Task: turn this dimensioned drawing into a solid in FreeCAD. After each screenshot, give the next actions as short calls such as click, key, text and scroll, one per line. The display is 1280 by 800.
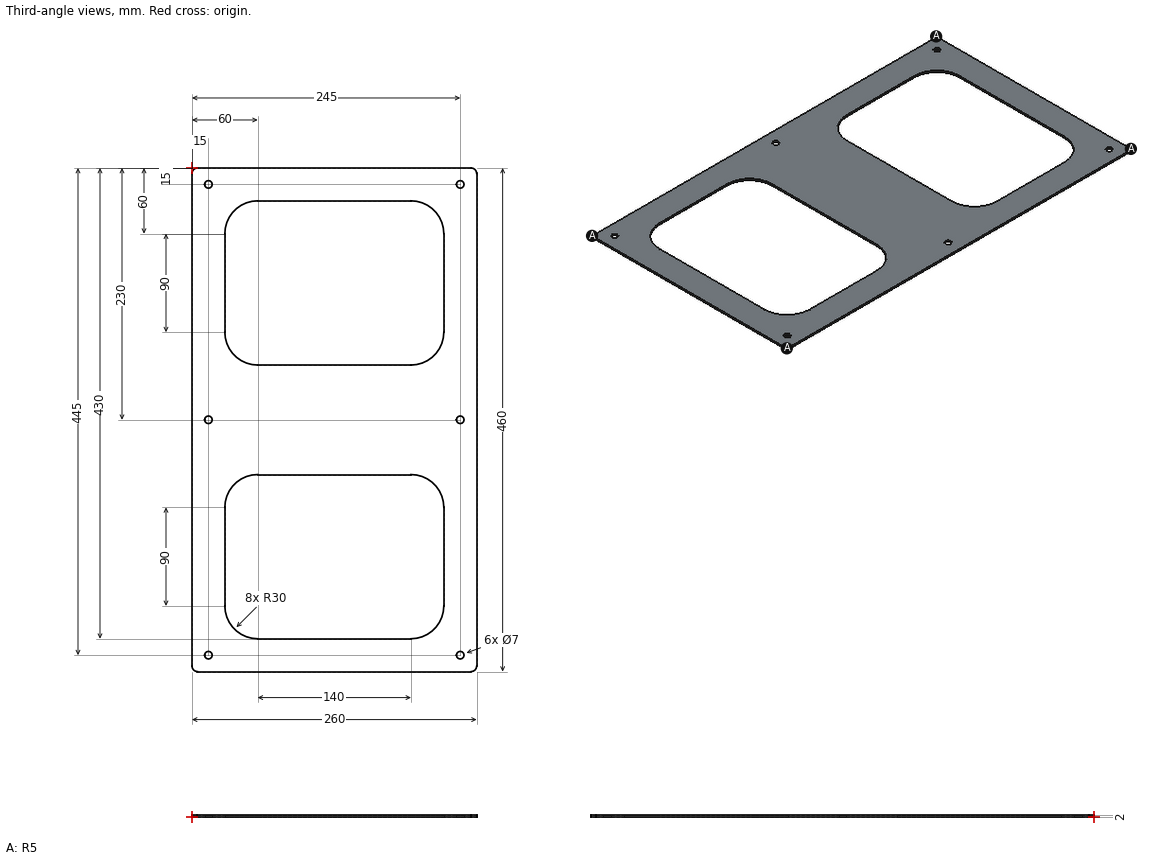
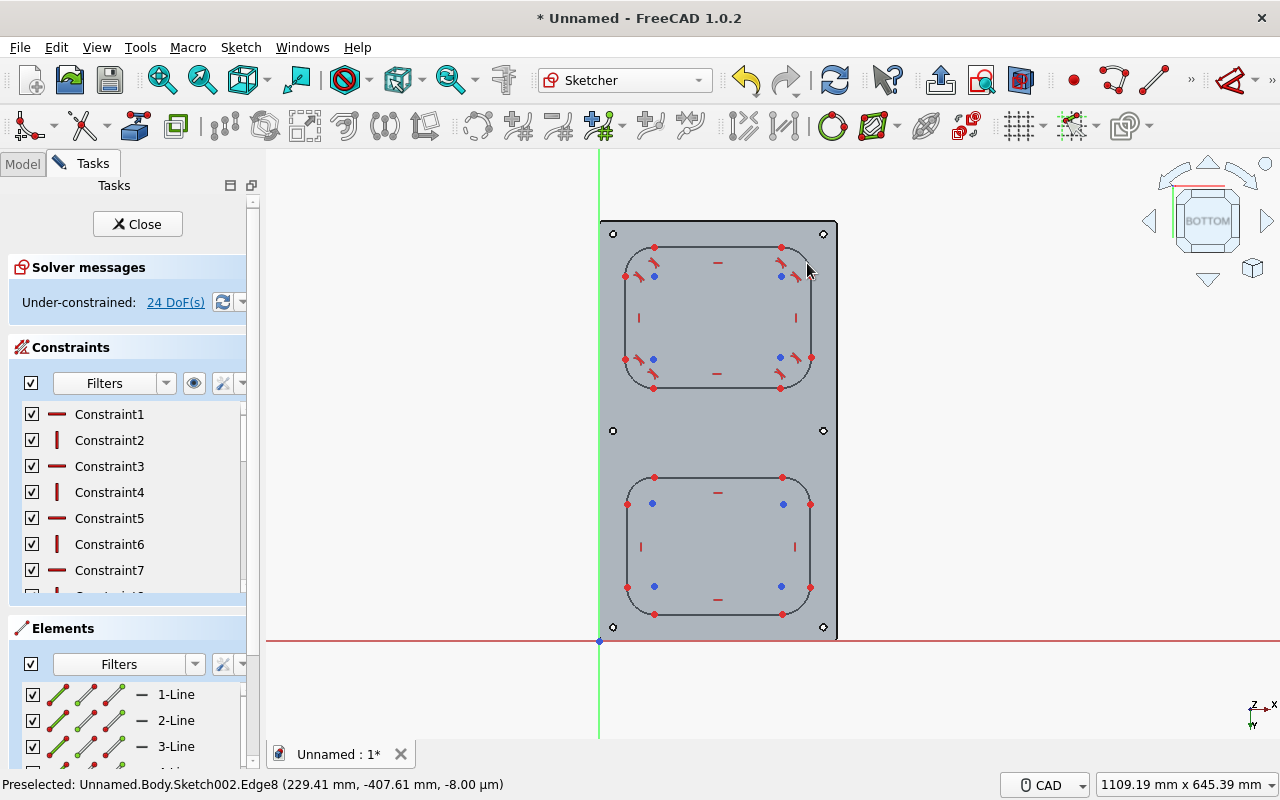
click(744, 478)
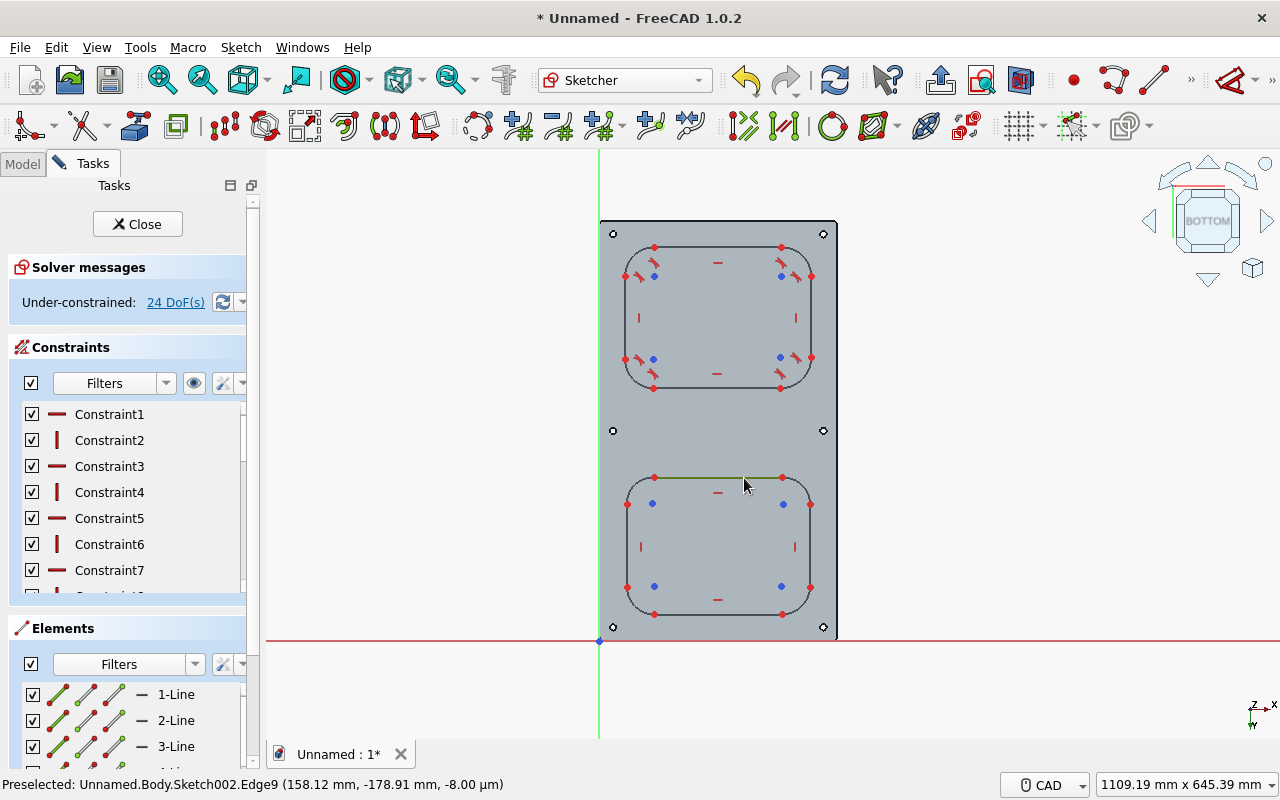
click(642, 480)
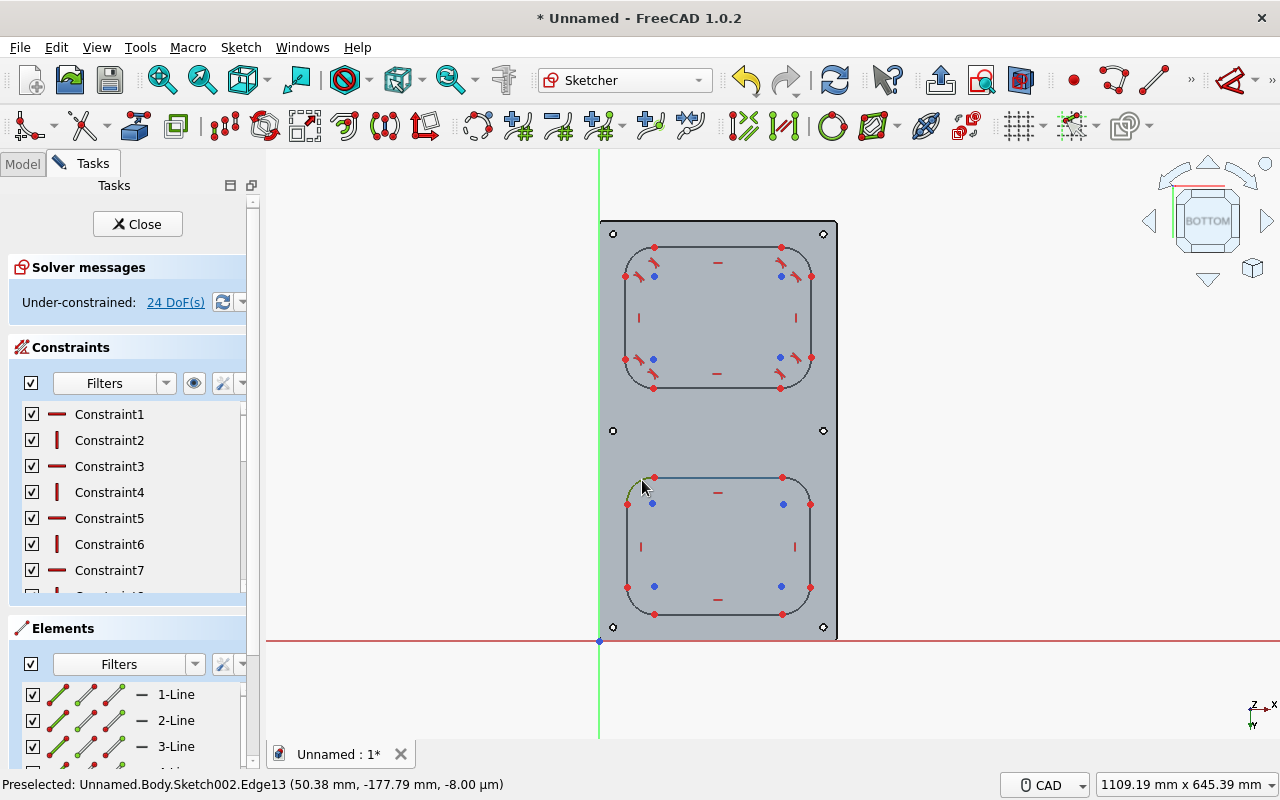
key(t)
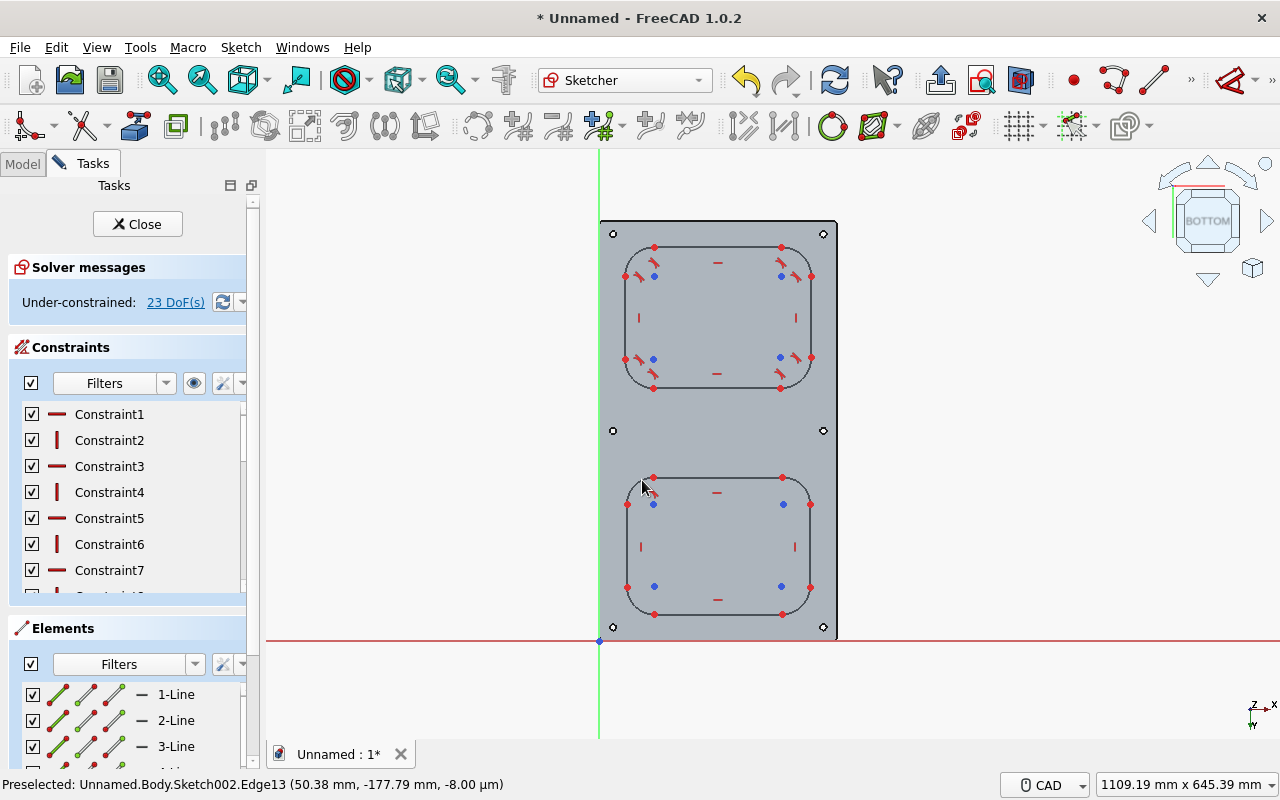
click(744, 478)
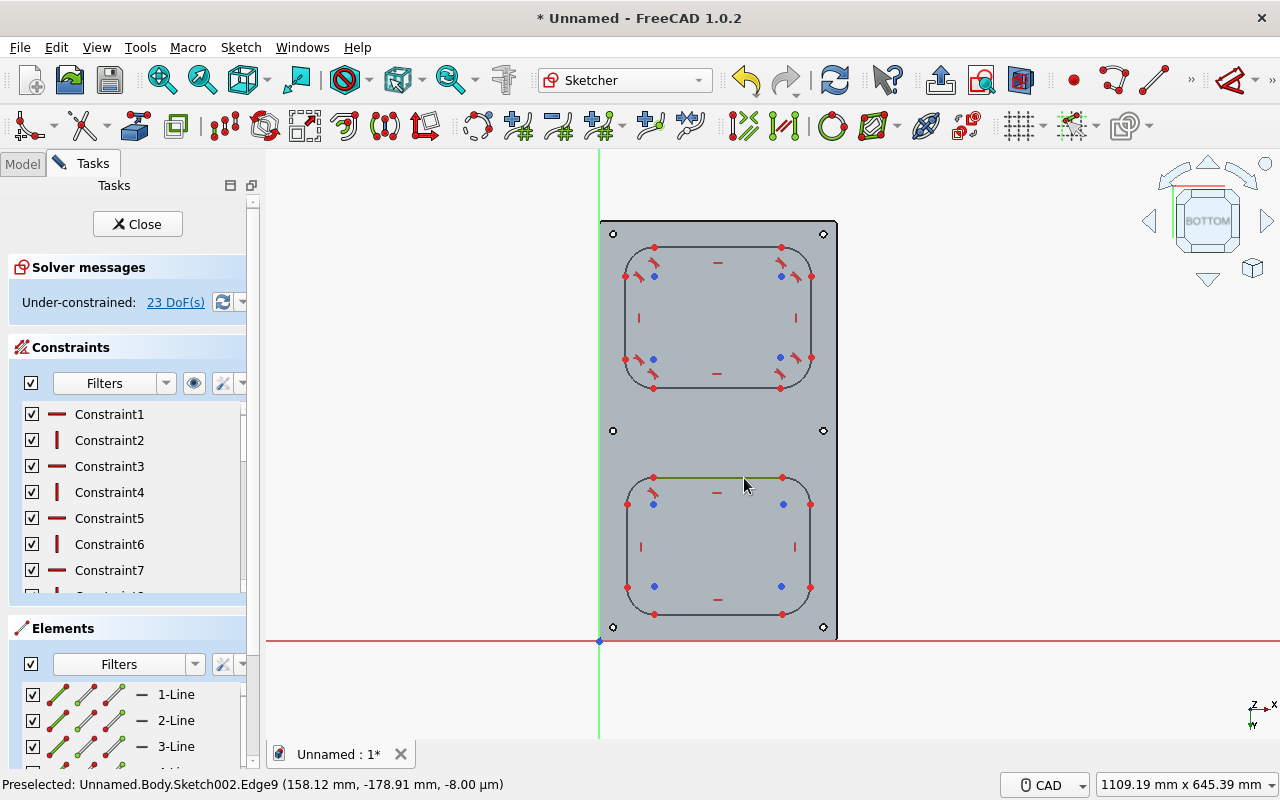
click(807, 492)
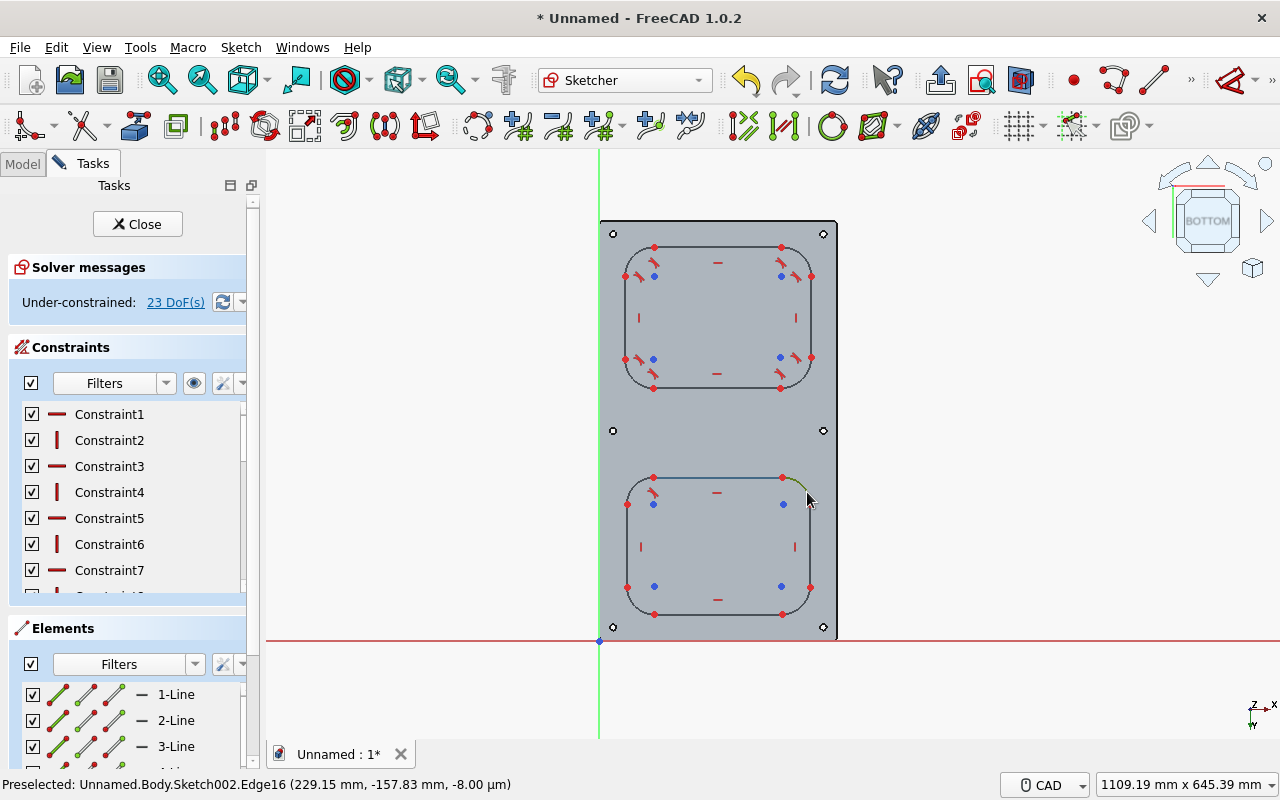
key(t)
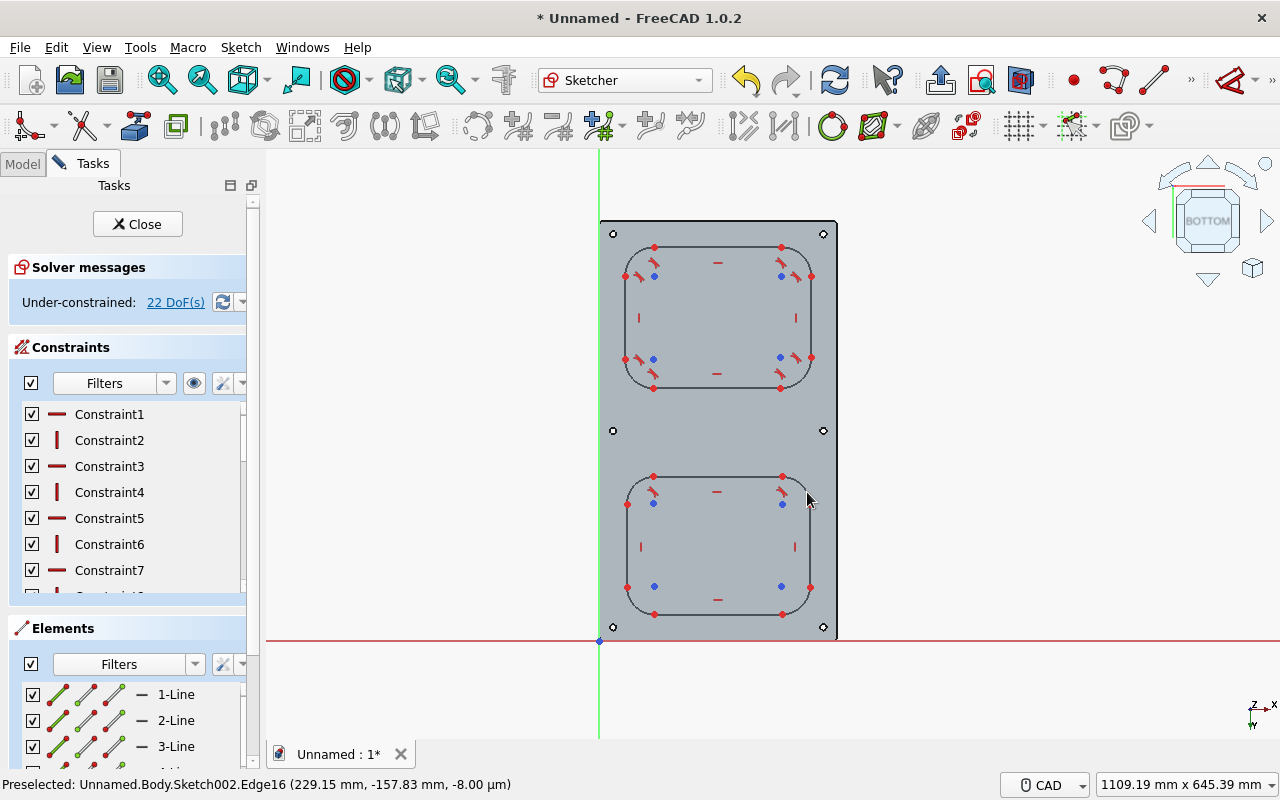
click(627, 529)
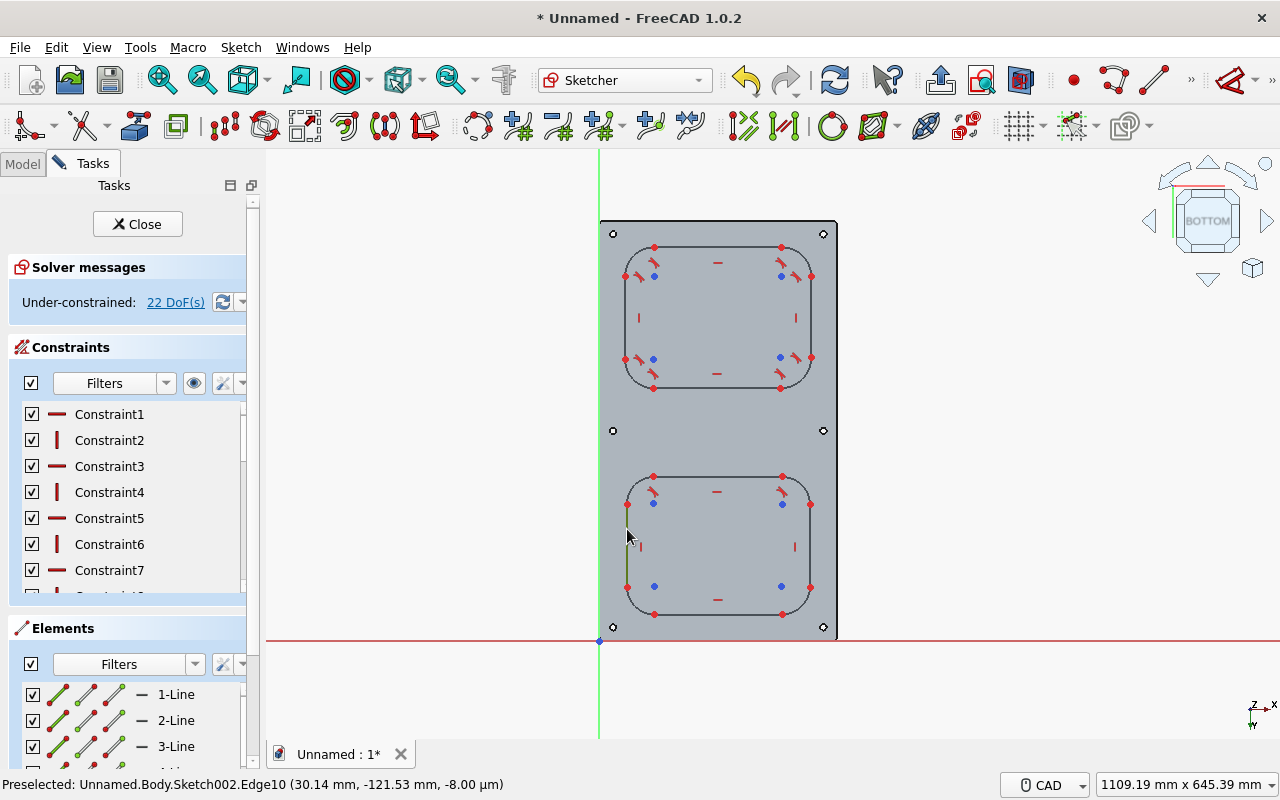
click(642, 480)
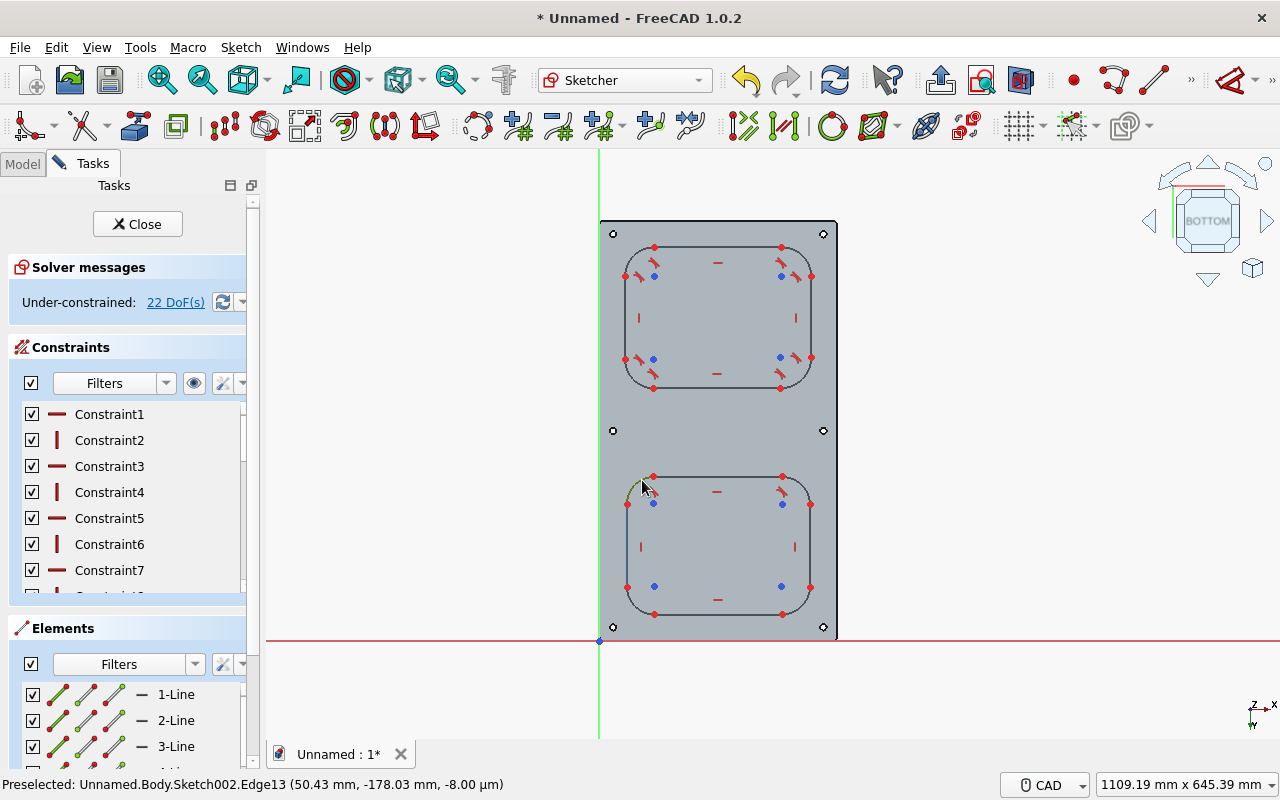
key(t)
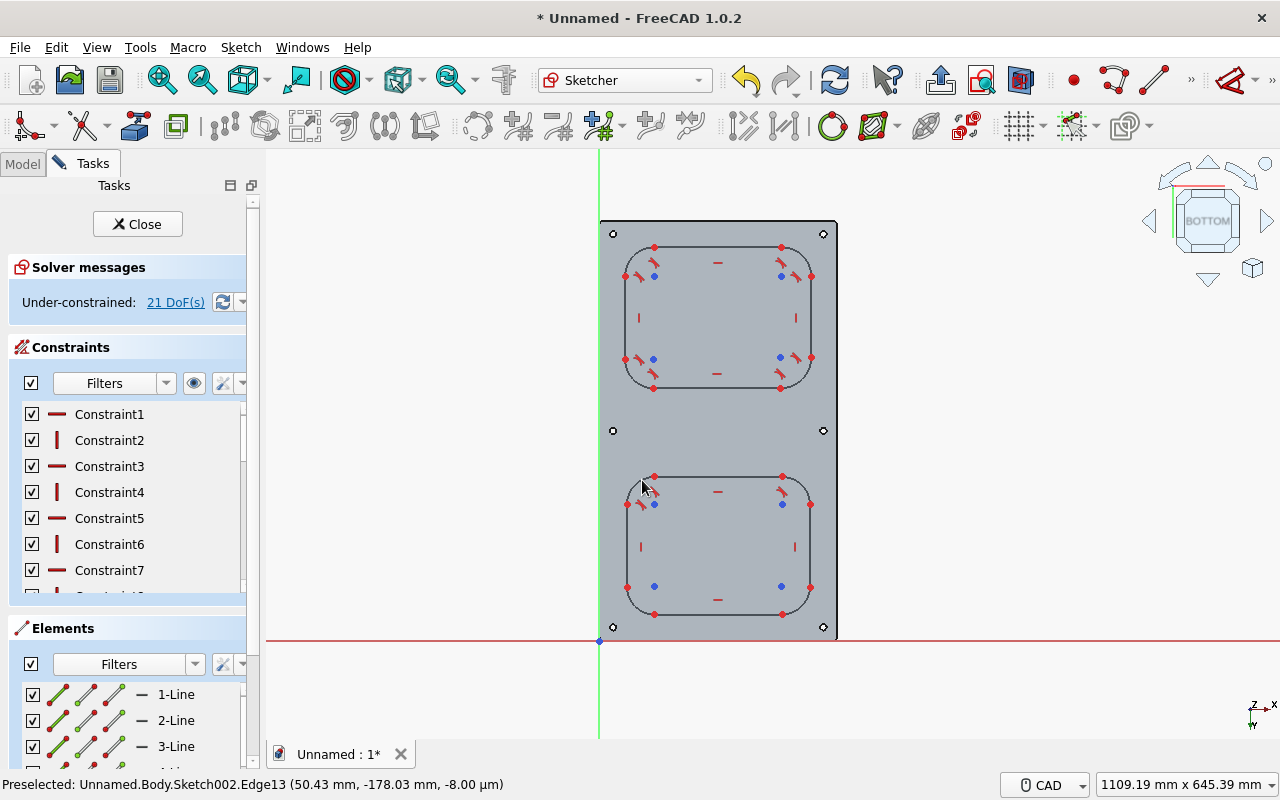
click(627, 529)